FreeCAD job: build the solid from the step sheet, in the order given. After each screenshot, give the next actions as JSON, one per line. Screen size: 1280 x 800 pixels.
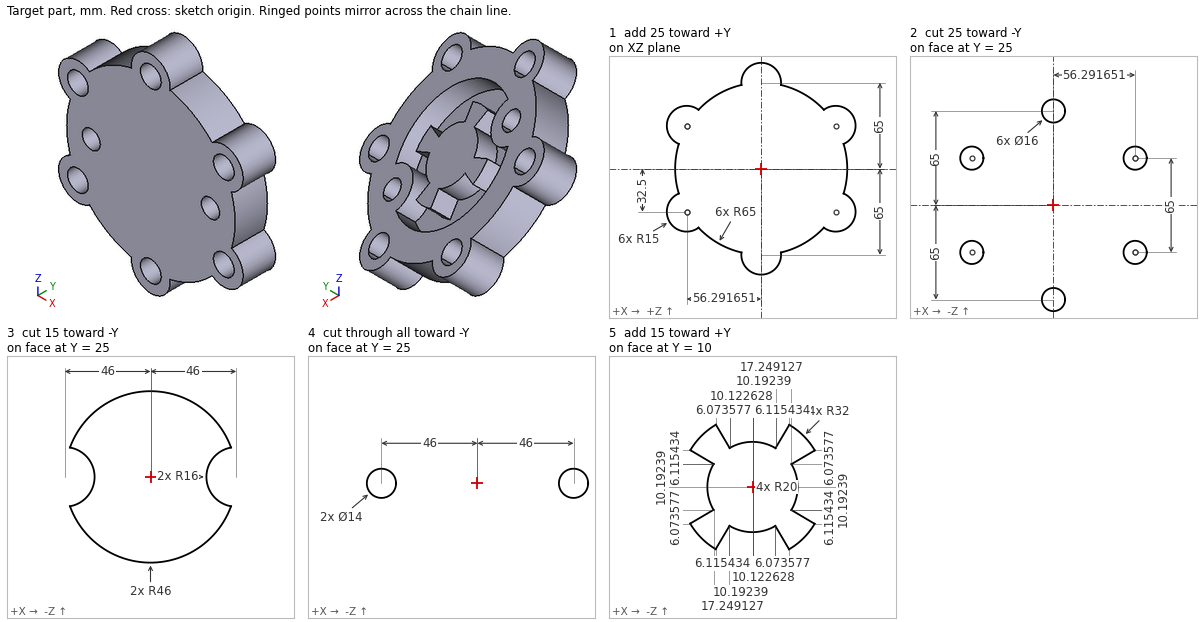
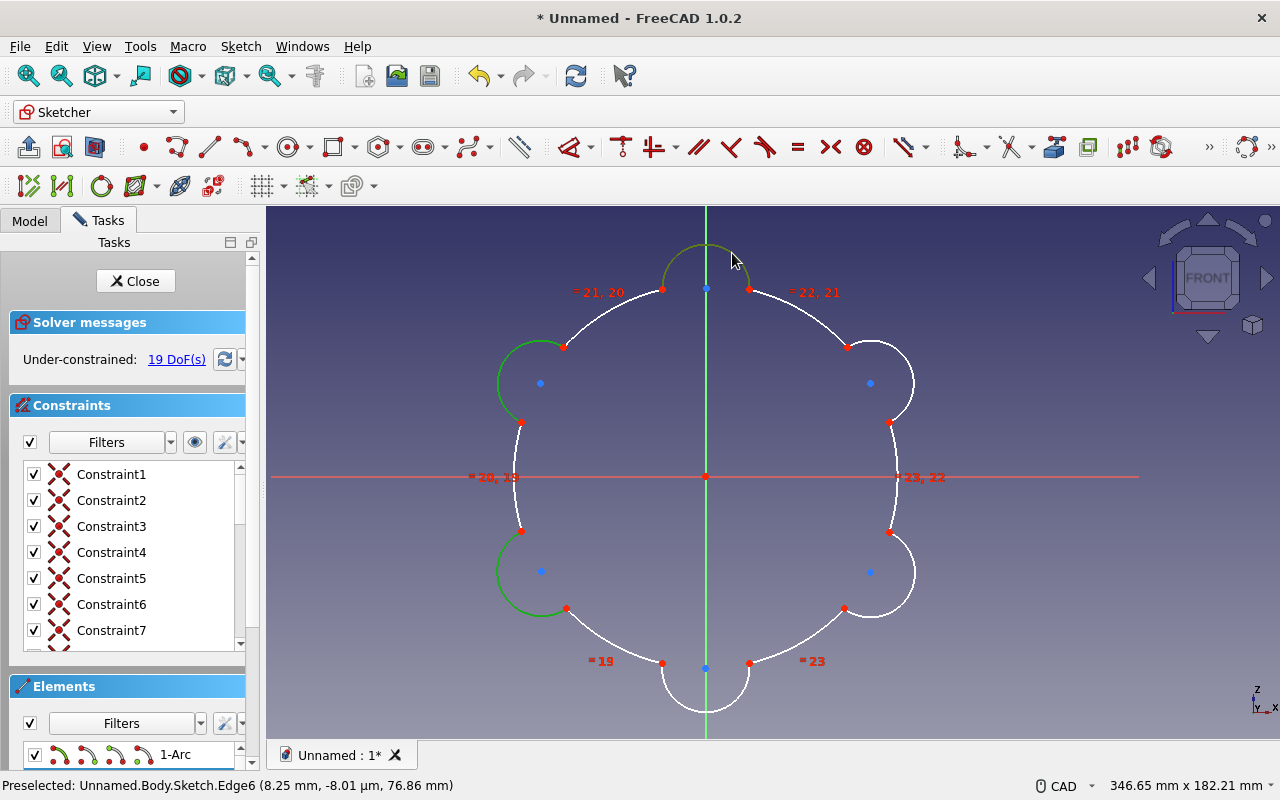
{"action": "left_click", "coordinate": [913, 389]}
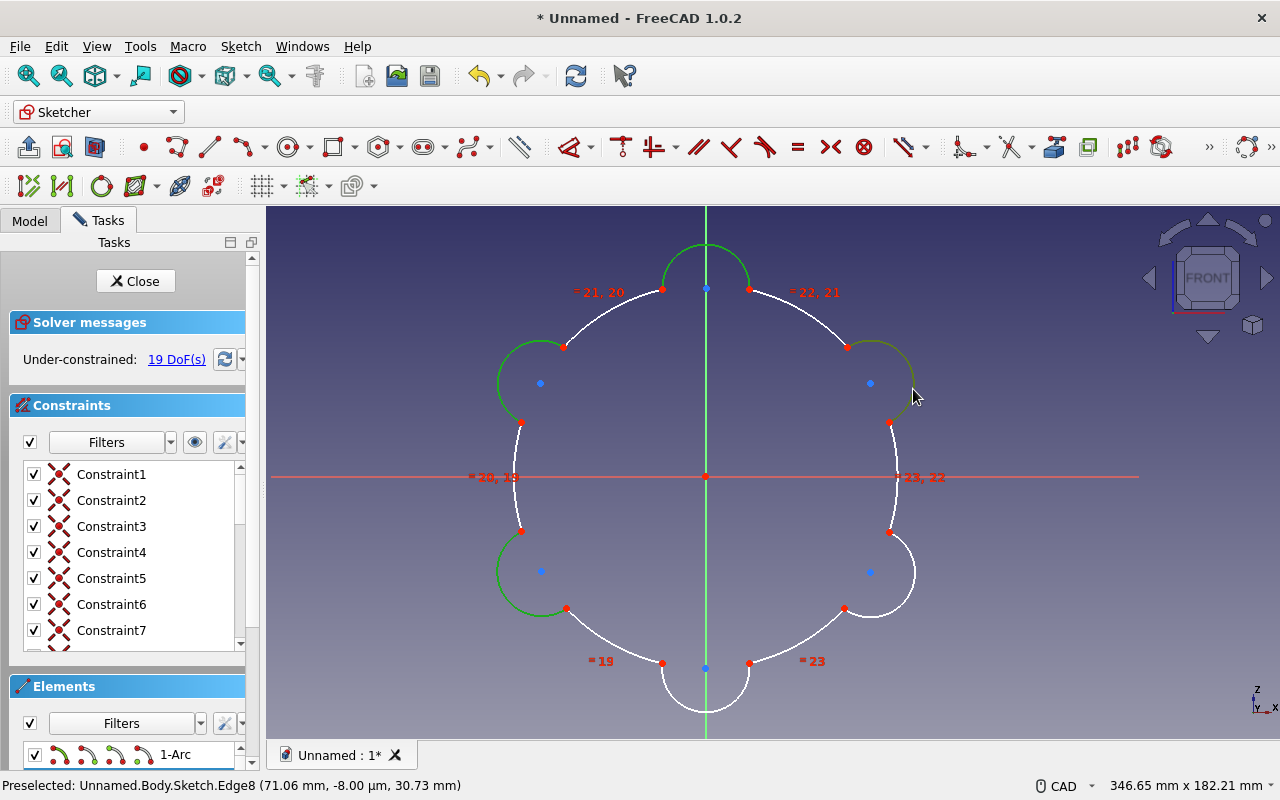
{"action": "left_click", "coordinate": [887, 614]}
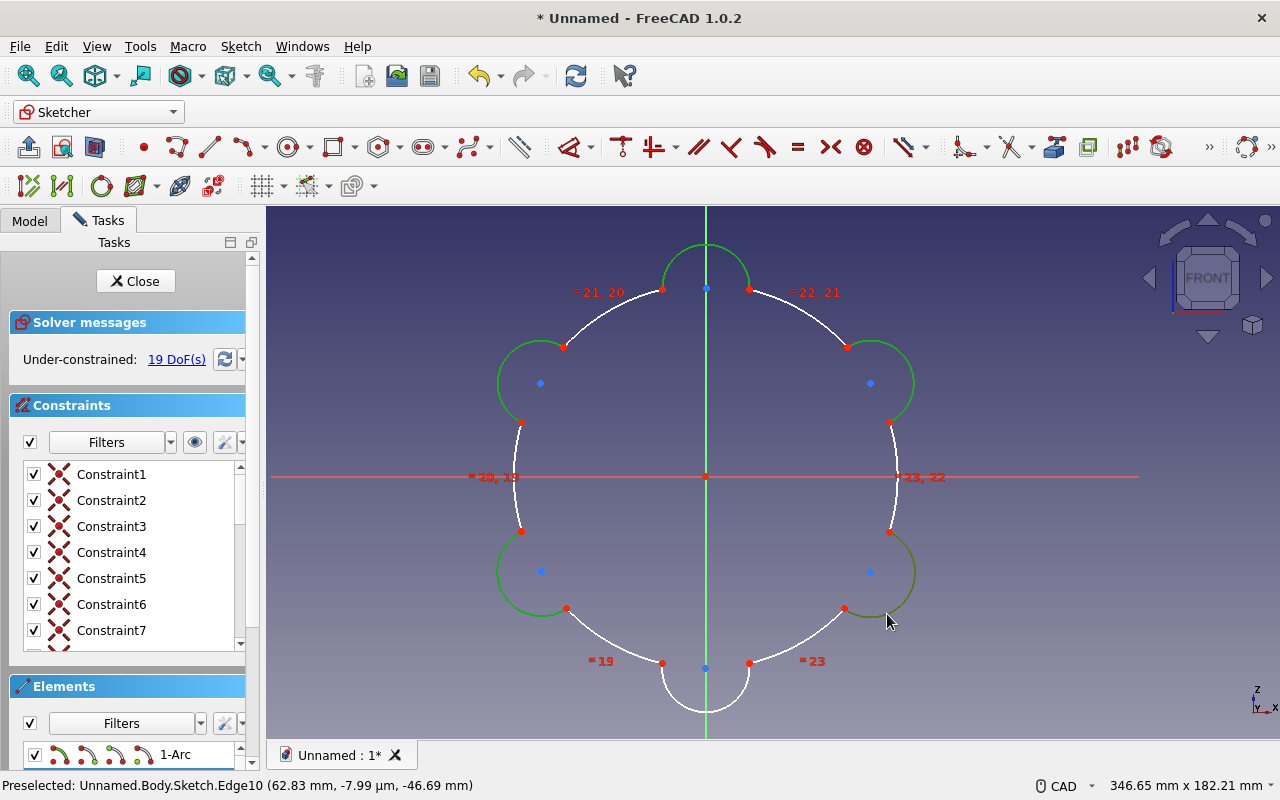
{"action": "left_click", "coordinate": [678, 703]}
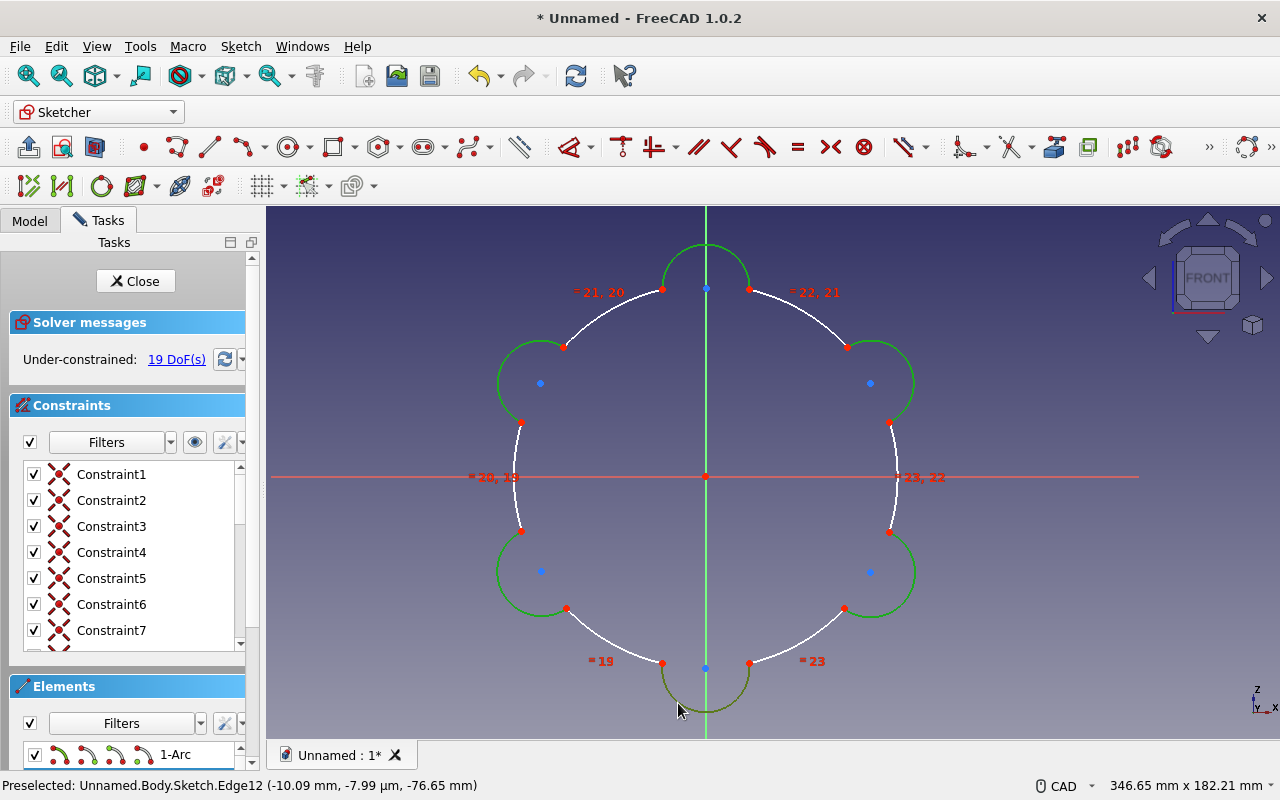
{"action": "left_click", "coordinate": [798, 148]}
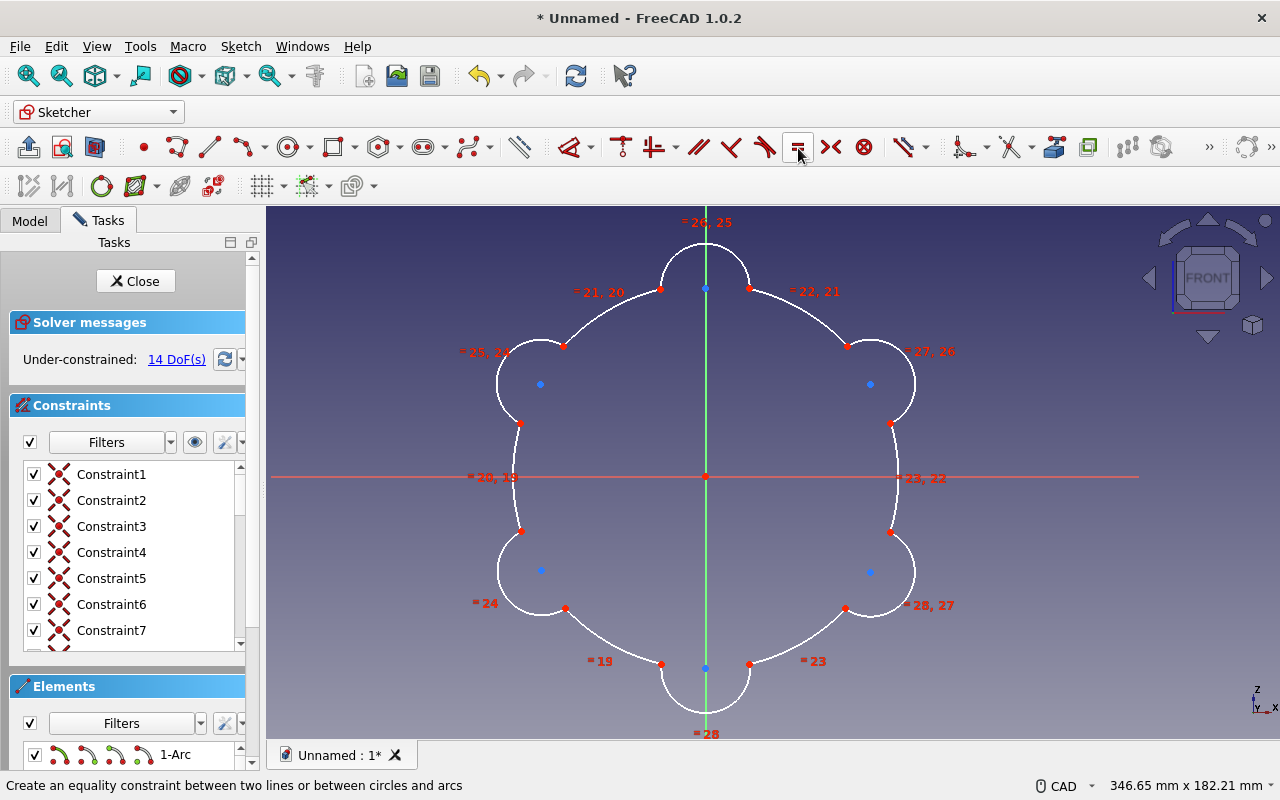
{"action": "left_click", "coordinate": [705, 288]}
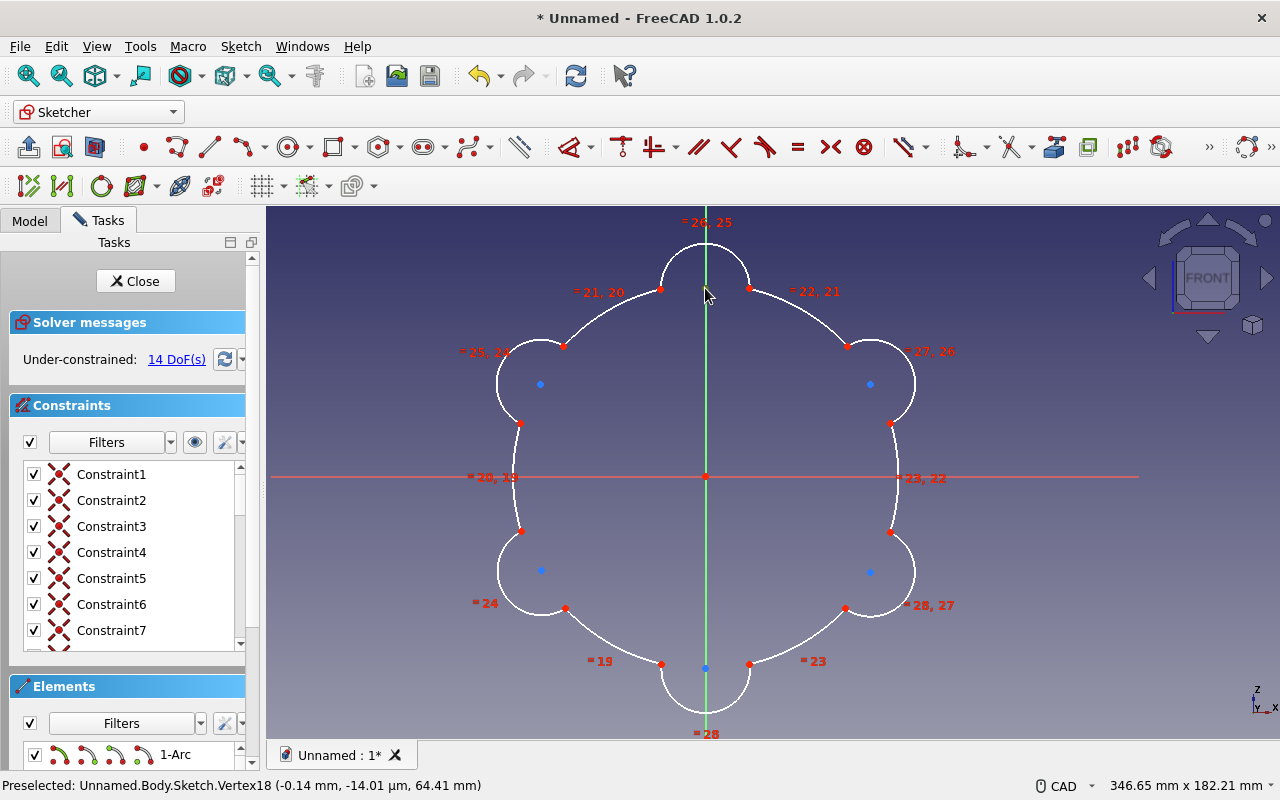
{"action": "left_click", "coordinate": [706, 677]}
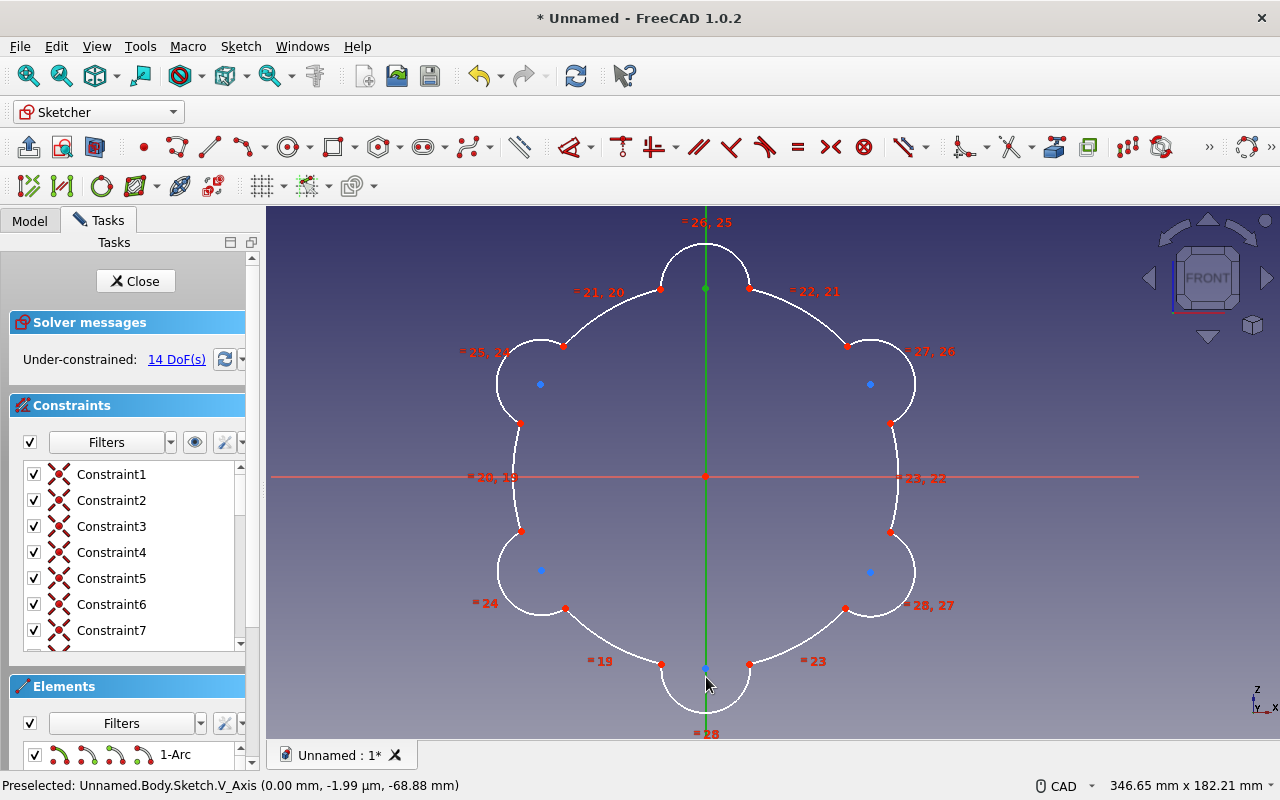
{"action": "left_click", "coordinate": [621, 148]}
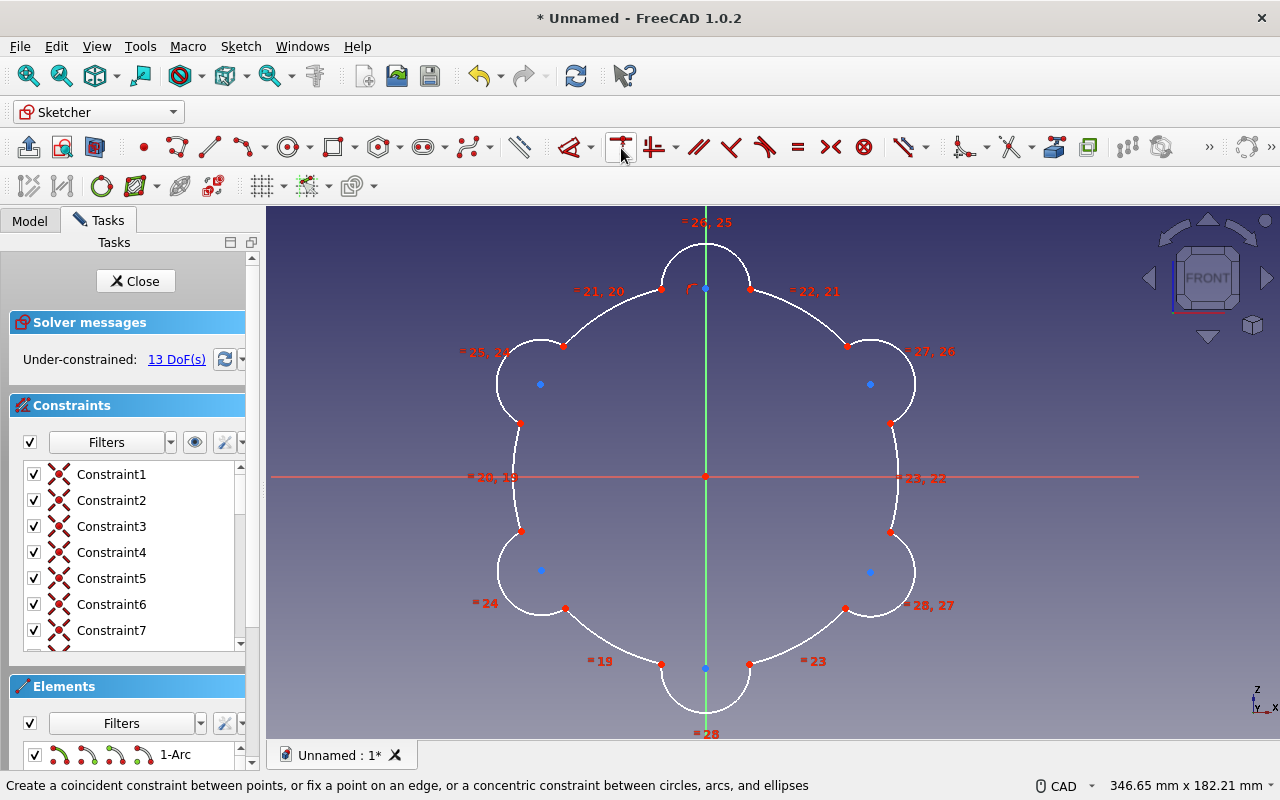
{"action": "left_click", "coordinate": [706, 669]}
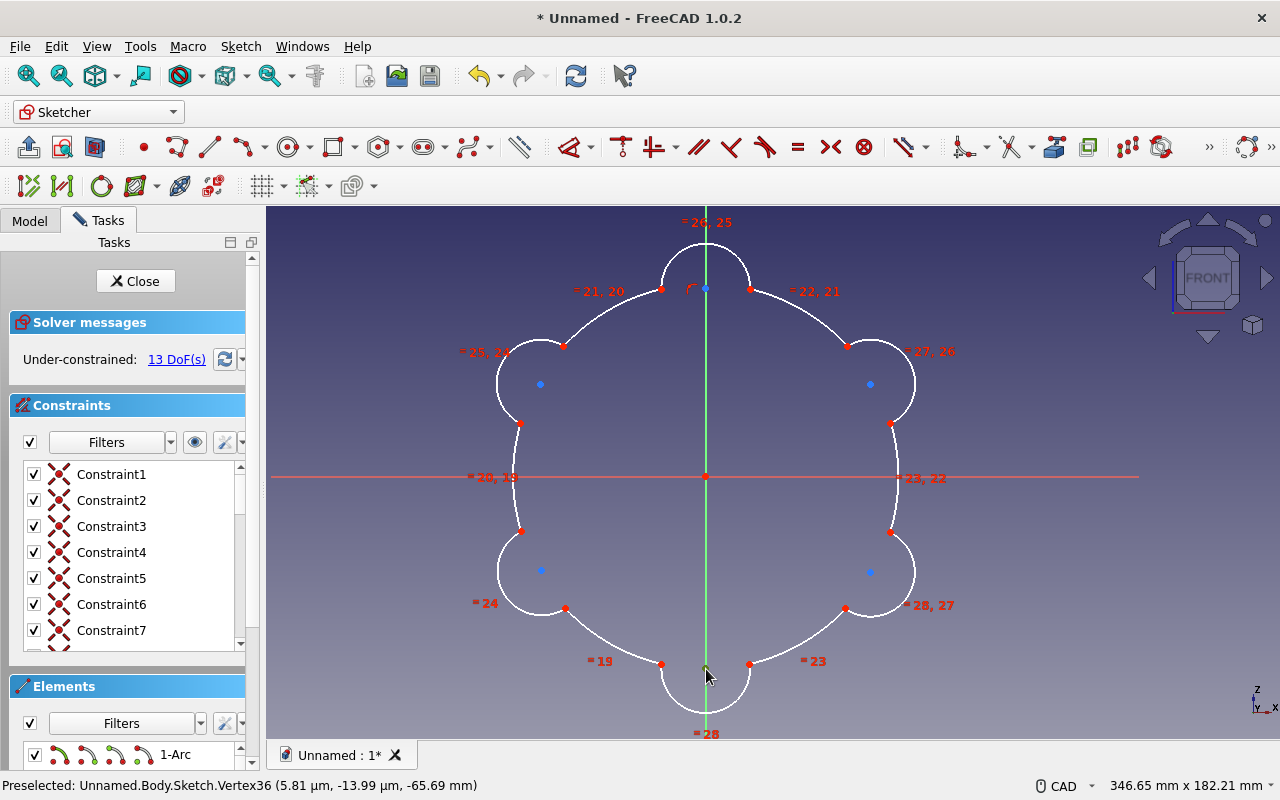
{"action": "left_click", "coordinate": [706, 677]}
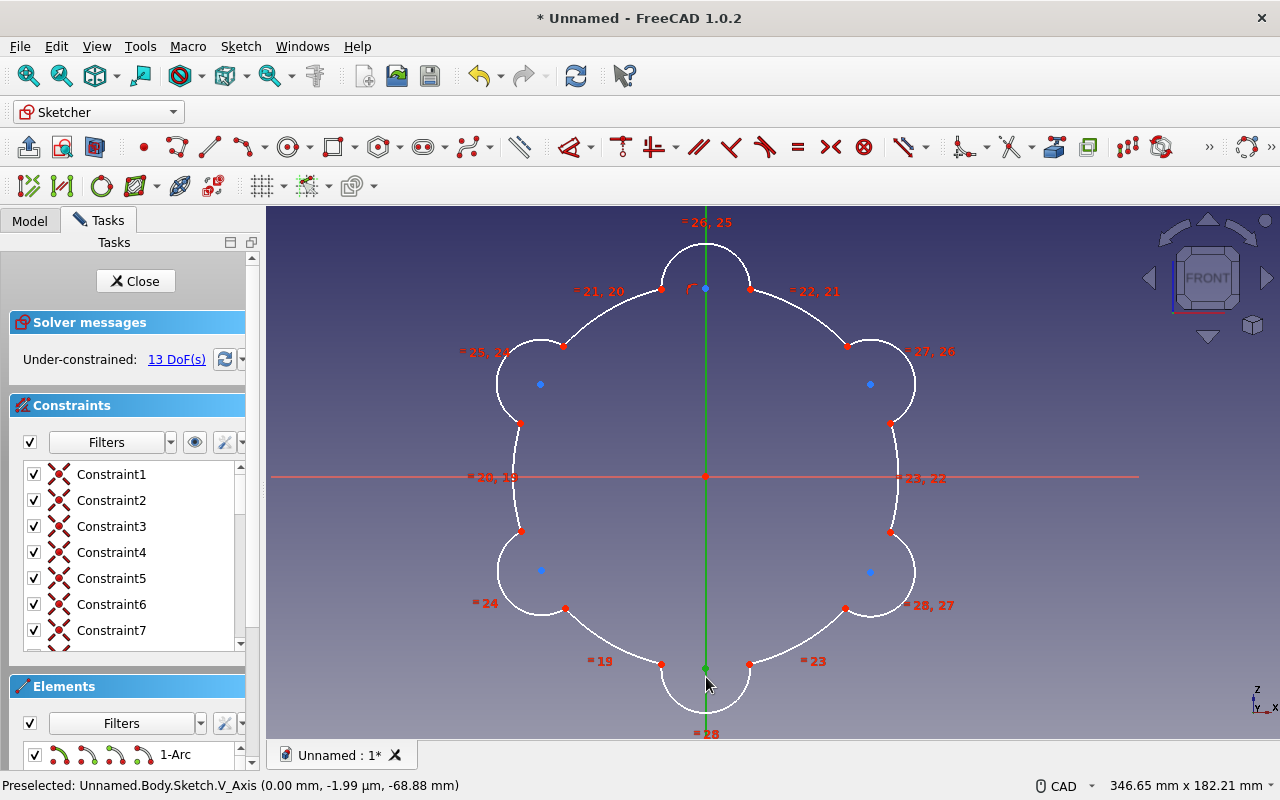
{"action": "left_click", "coordinate": [621, 148]}